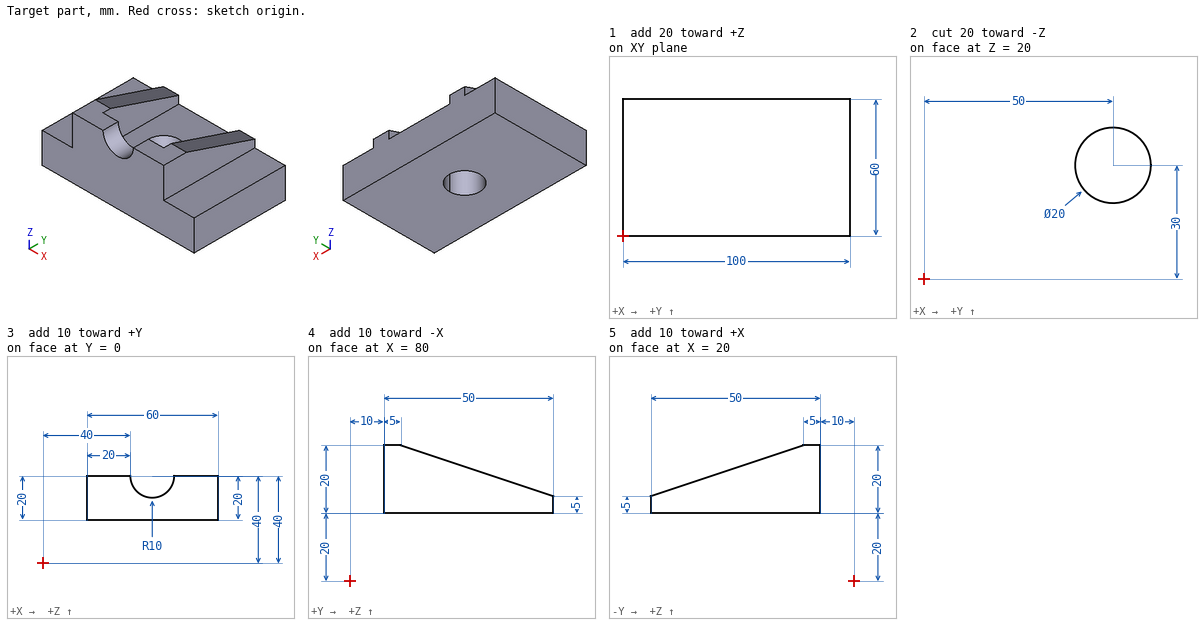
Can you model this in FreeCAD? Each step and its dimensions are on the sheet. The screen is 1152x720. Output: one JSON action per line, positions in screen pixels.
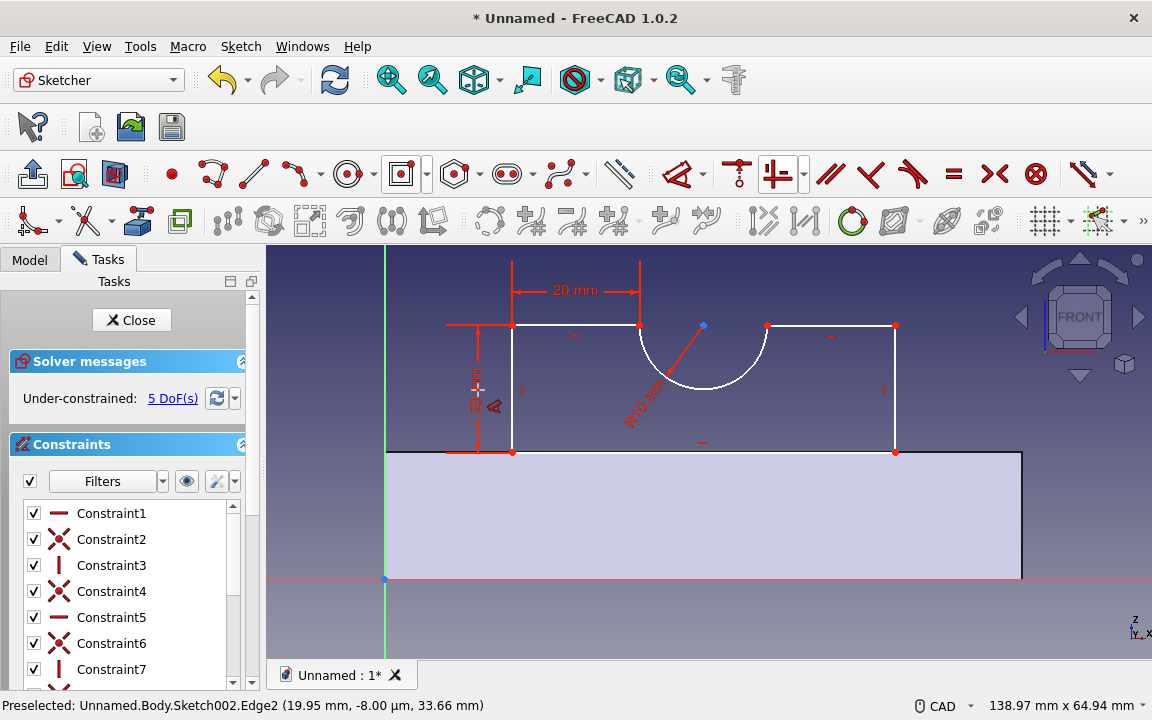
{"action": "left_click", "coordinate": [627, 453]}
{"action": "left_click", "coordinate": [704, 487]}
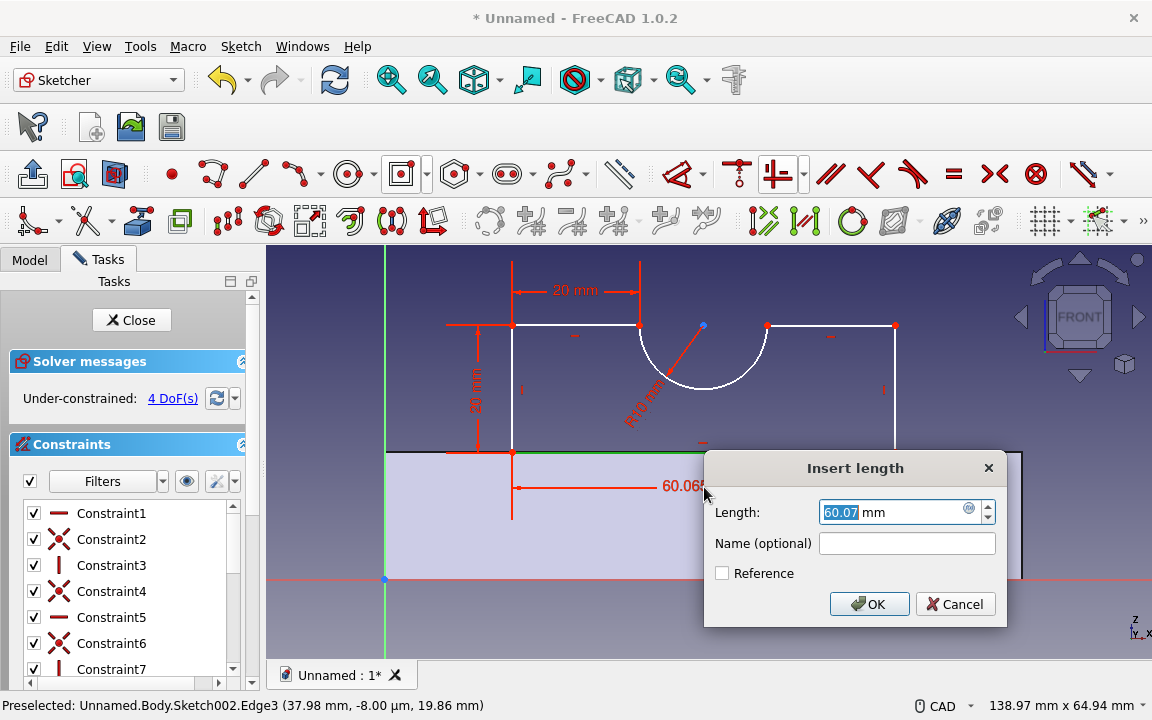
{"action": "type", "text": "60"}
{"action": "key", "text": "Return"}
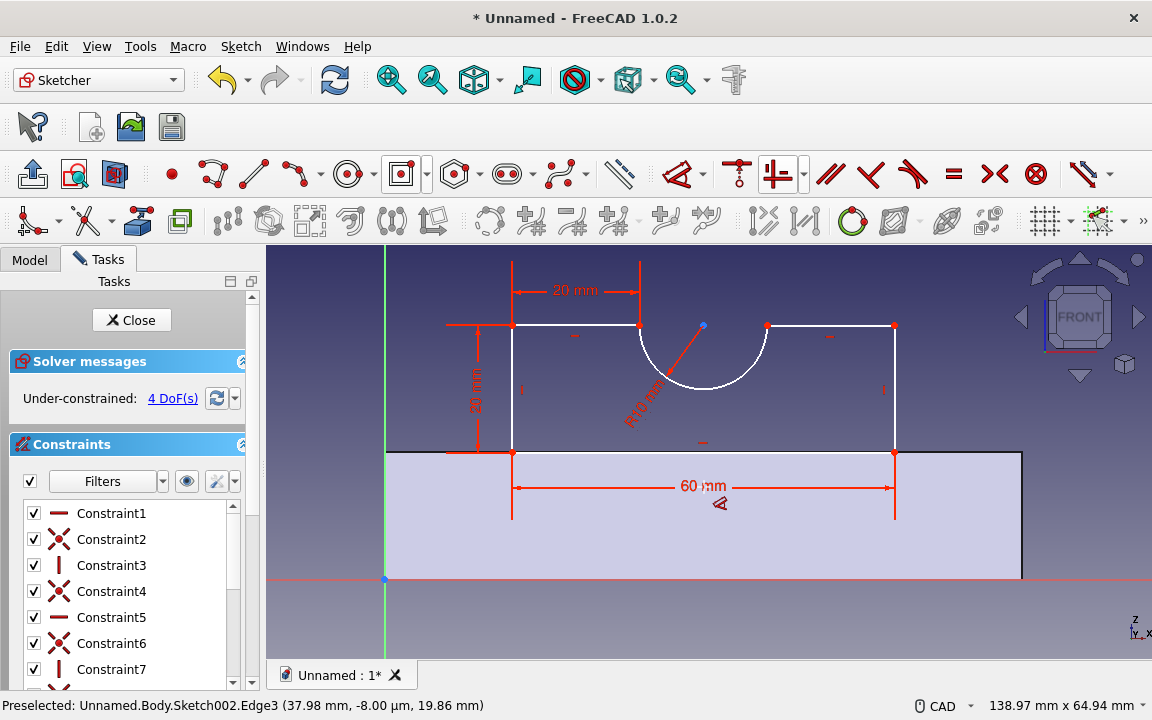
{"action": "left_click", "coordinate": [895, 415]}
{"action": "left_click", "coordinate": [929, 390]}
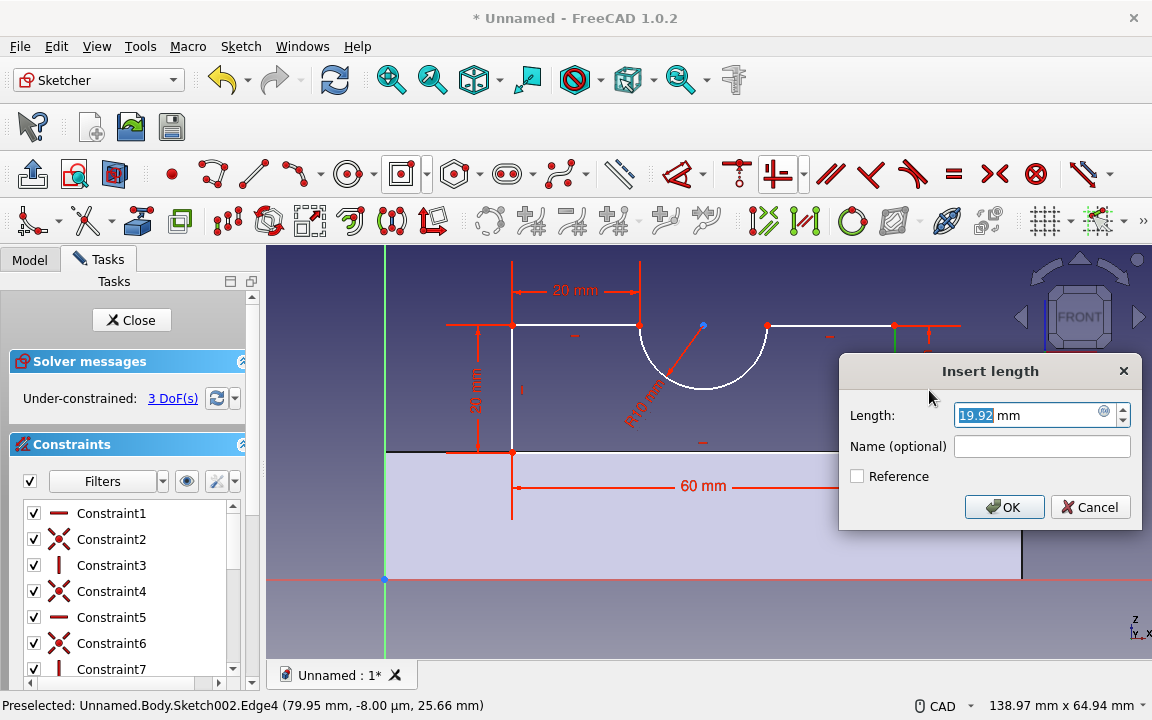
{"action": "type", "text": "20"}
{"action": "key", "text": "Return"}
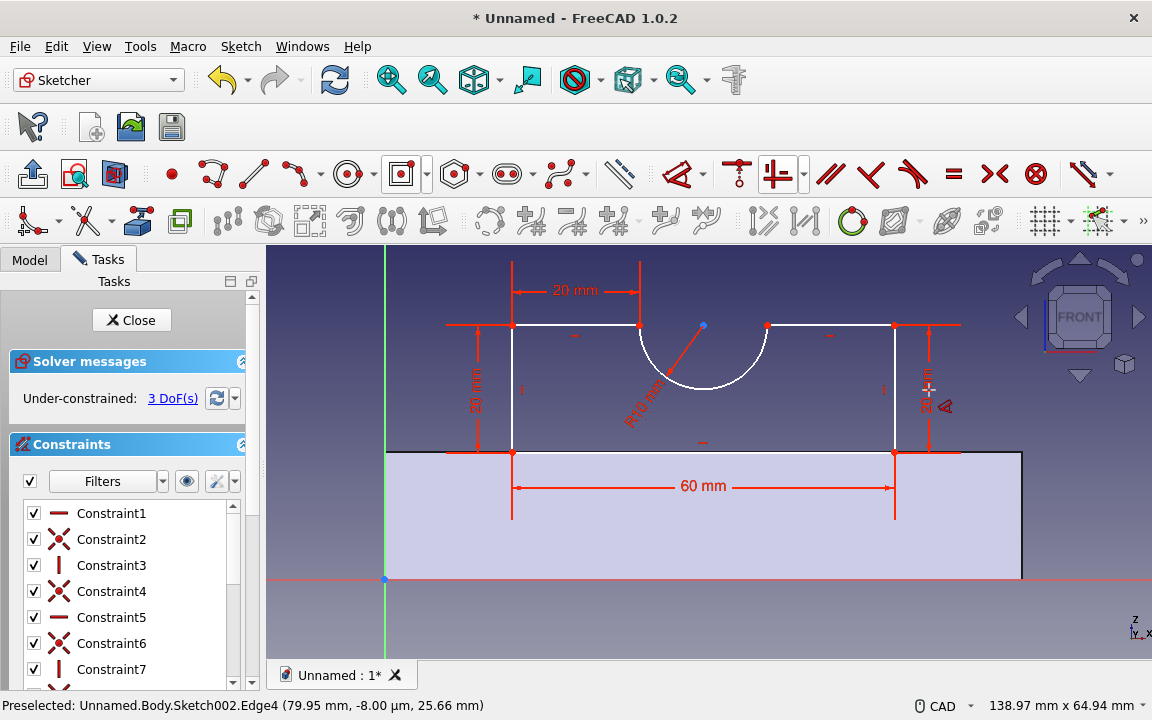
{"action": "left_click", "coordinate": [640, 325]}
{"action": "left_click", "coordinate": [512, 614]}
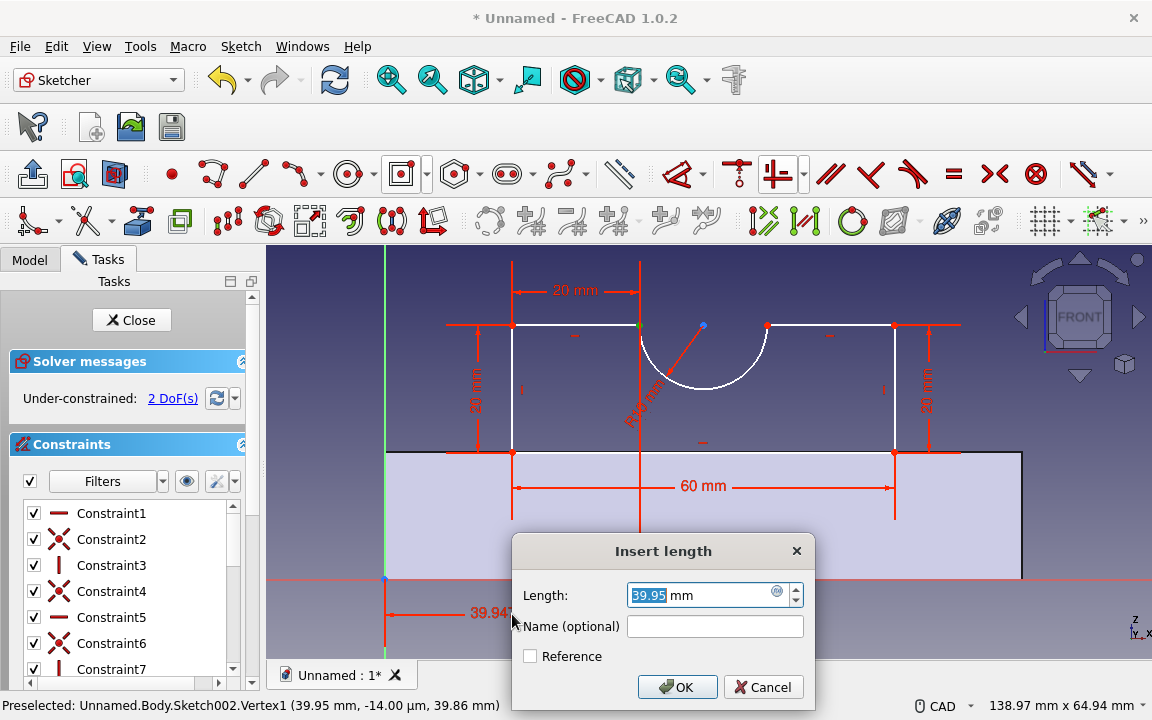
{"action": "type", "text": "40"}
{"action": "key", "text": "Return"}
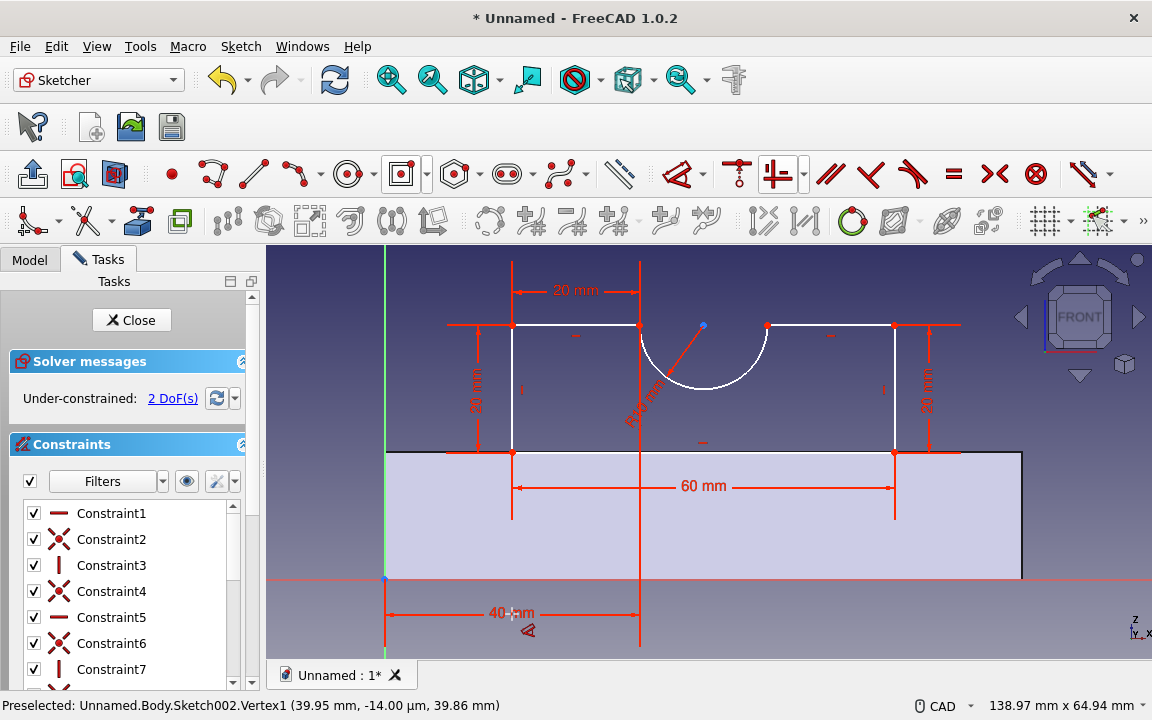
{"action": "left_click", "coordinate": [640, 325]}
{"action": "left_click", "coordinate": [351, 453]}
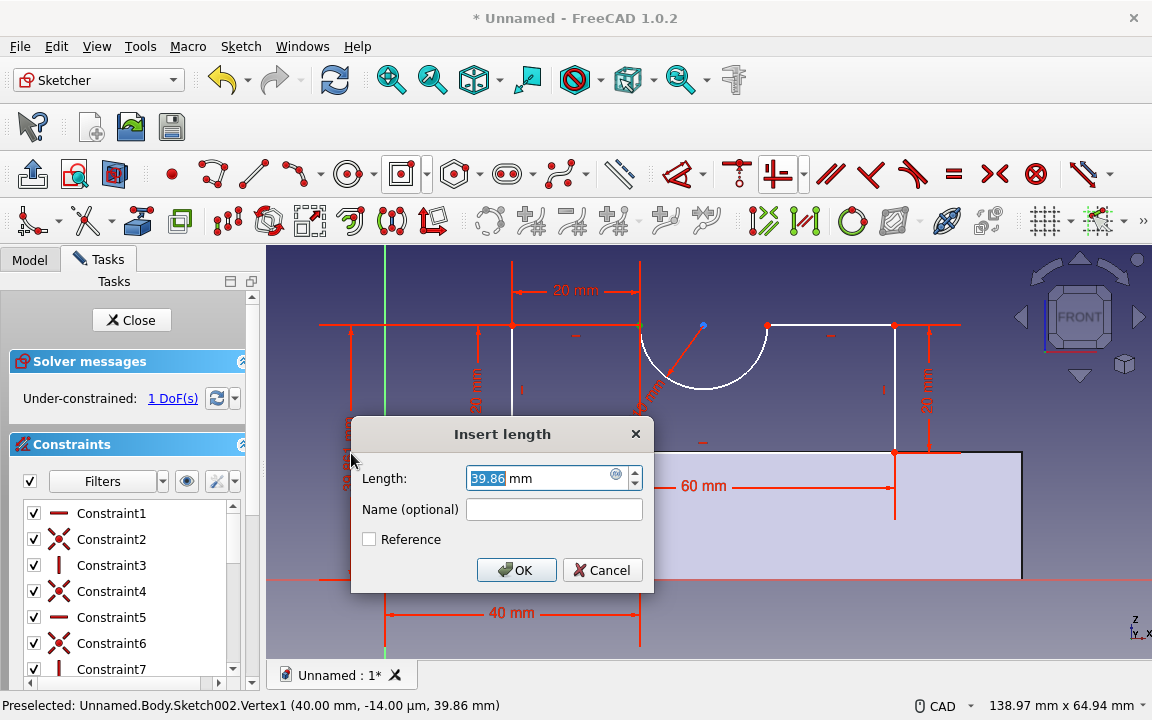
{"action": "type", "text": "40"}
{"action": "key", "text": "Return"}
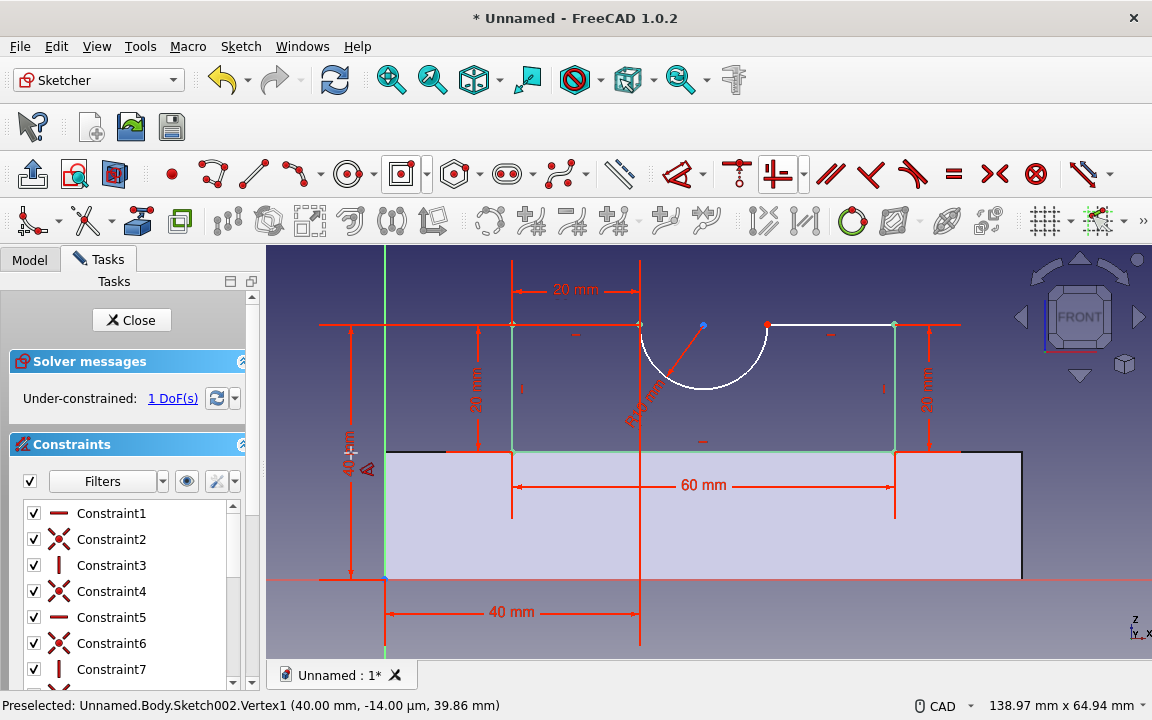
{"action": "left_click", "coordinate": [704, 325]}
{"action": "left_click", "coordinate": [351, 394]}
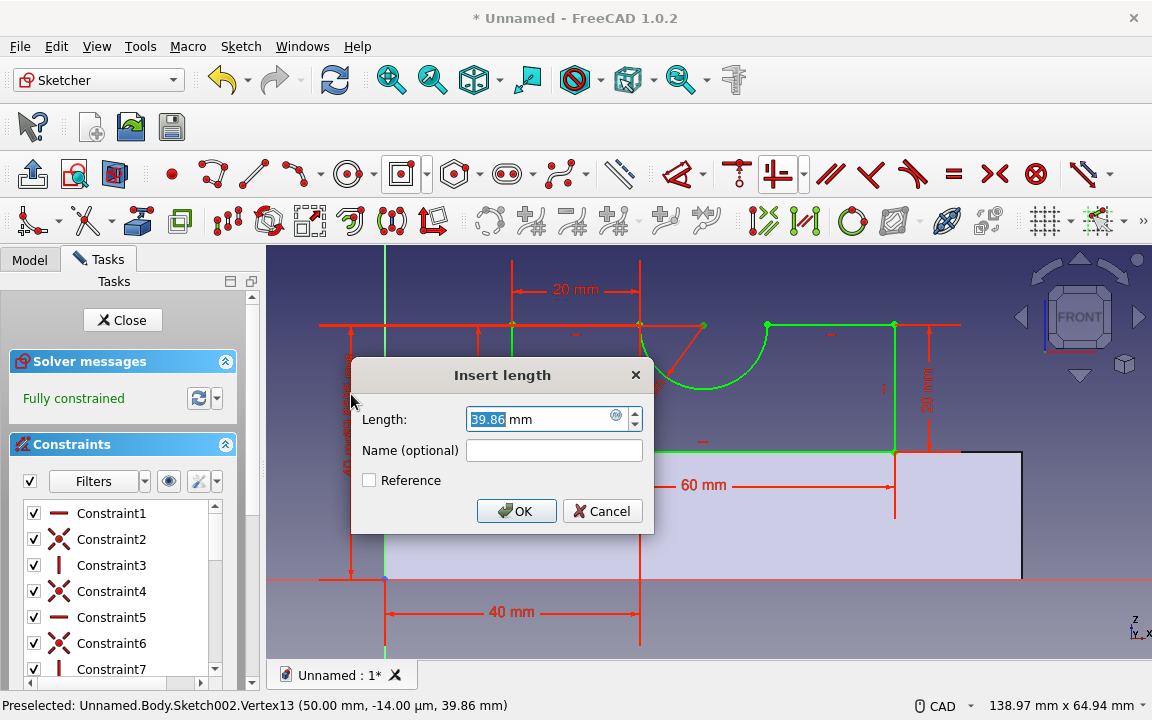
{"action": "type", "text": "40"}
{"action": "key", "text": "Return"}
{"action": "key", "text": "Escape"}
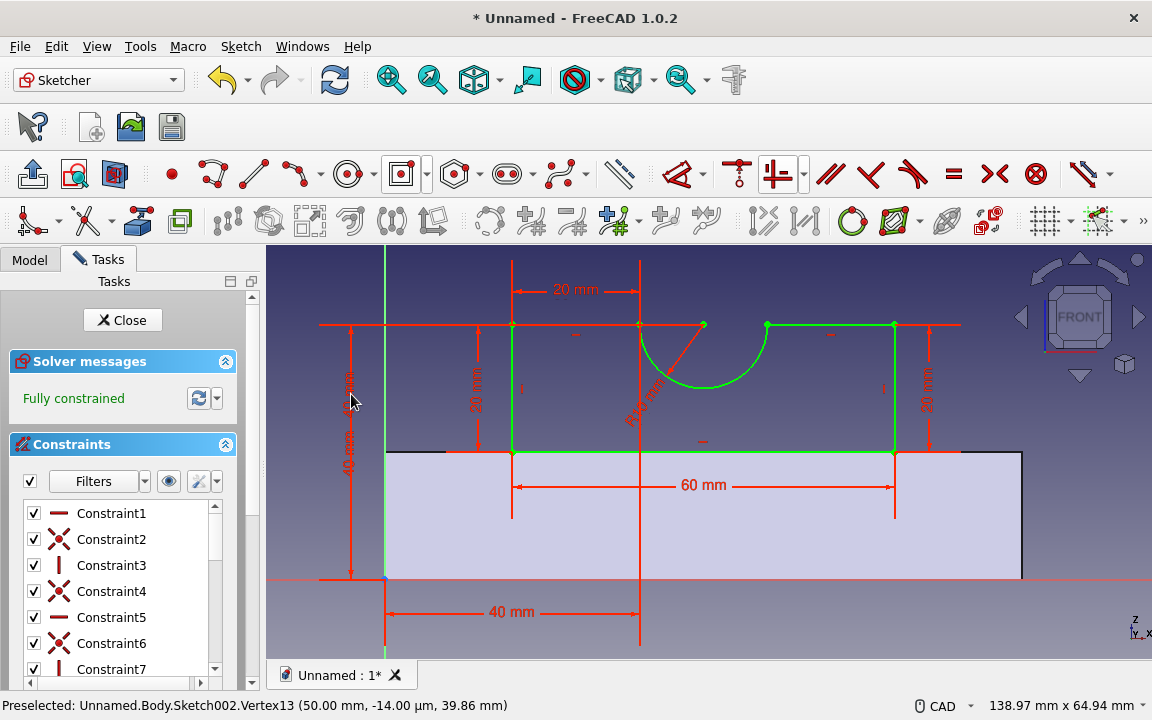
{"action": "left_click", "coordinate": [123, 320]}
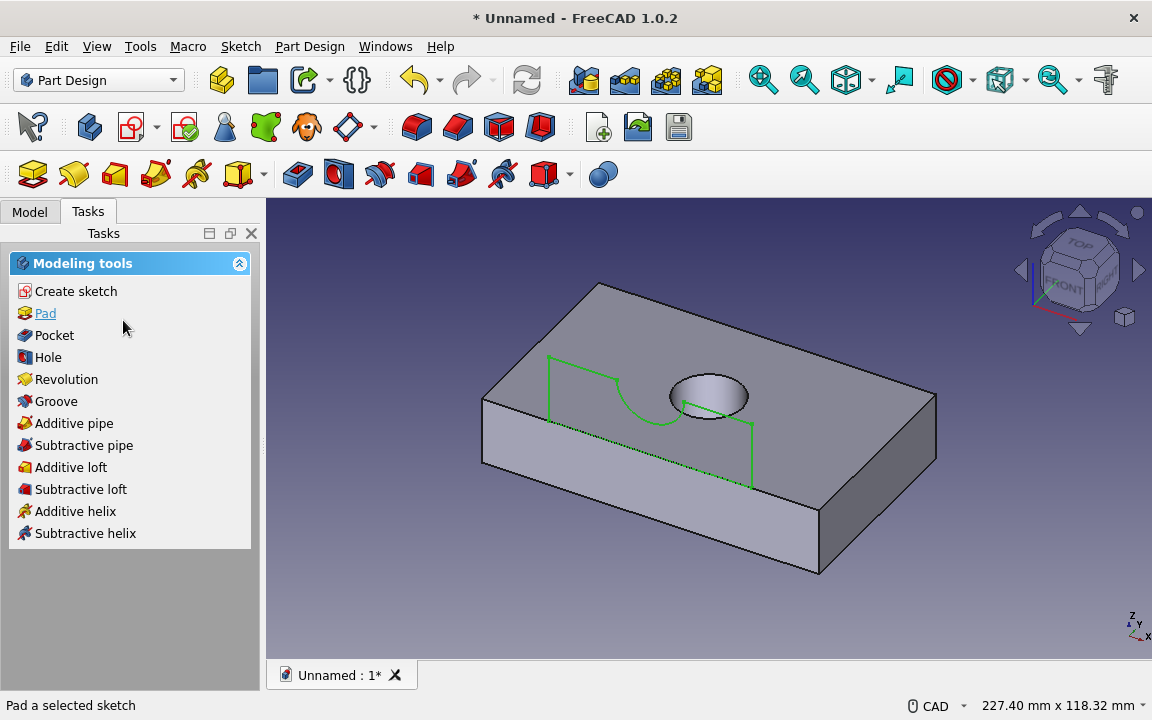
{"action": "left_click", "coordinate": [33, 174]}